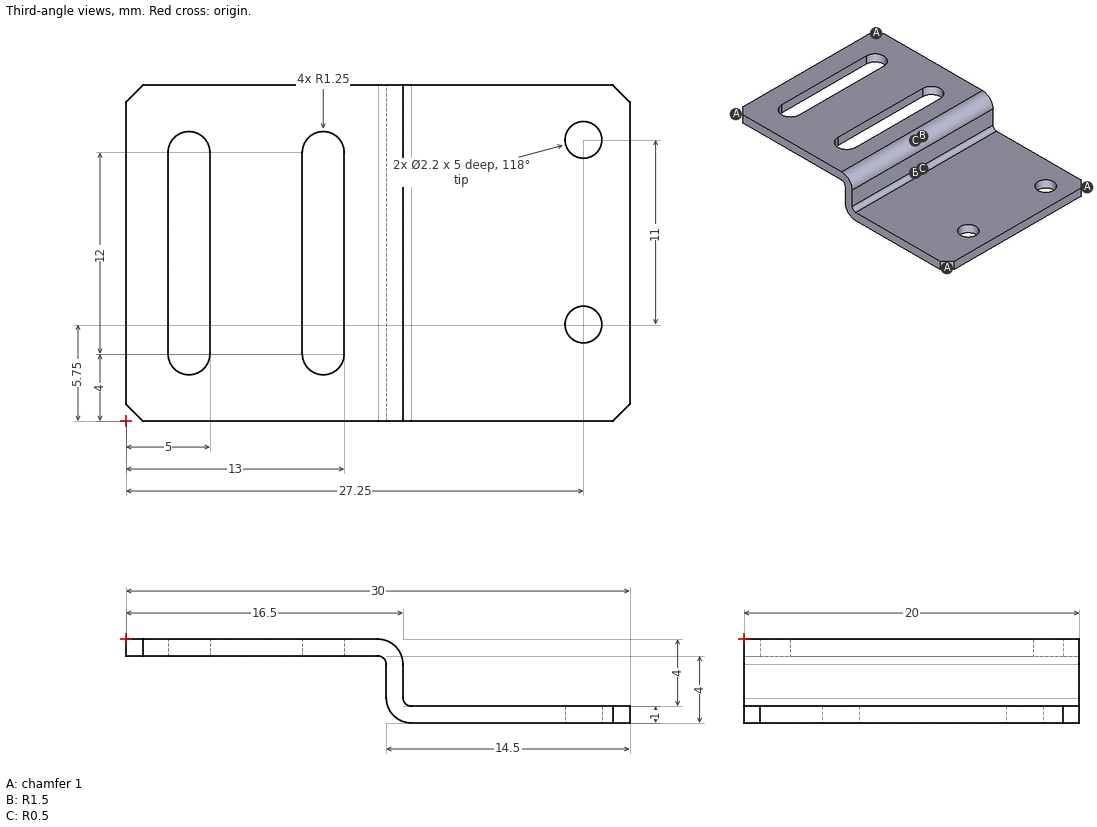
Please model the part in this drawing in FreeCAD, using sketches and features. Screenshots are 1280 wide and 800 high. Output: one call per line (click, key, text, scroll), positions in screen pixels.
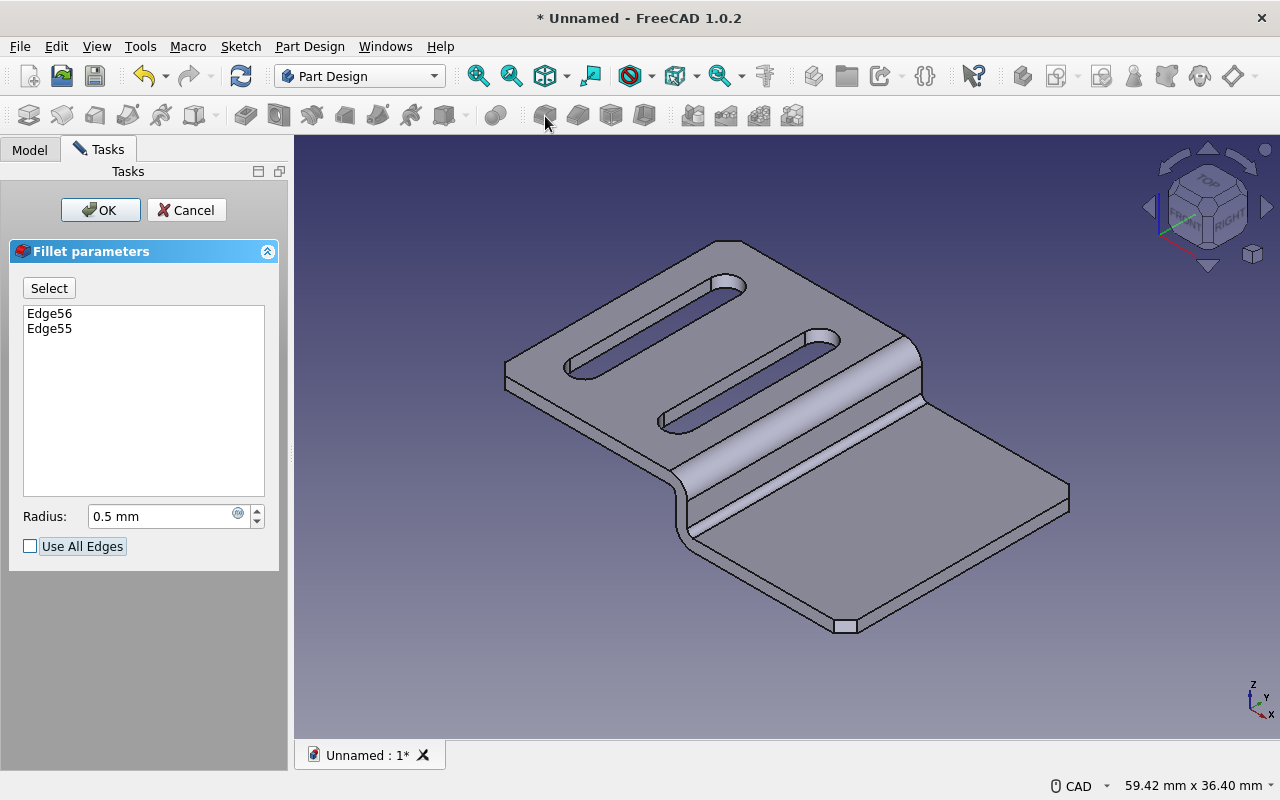
click(101, 210)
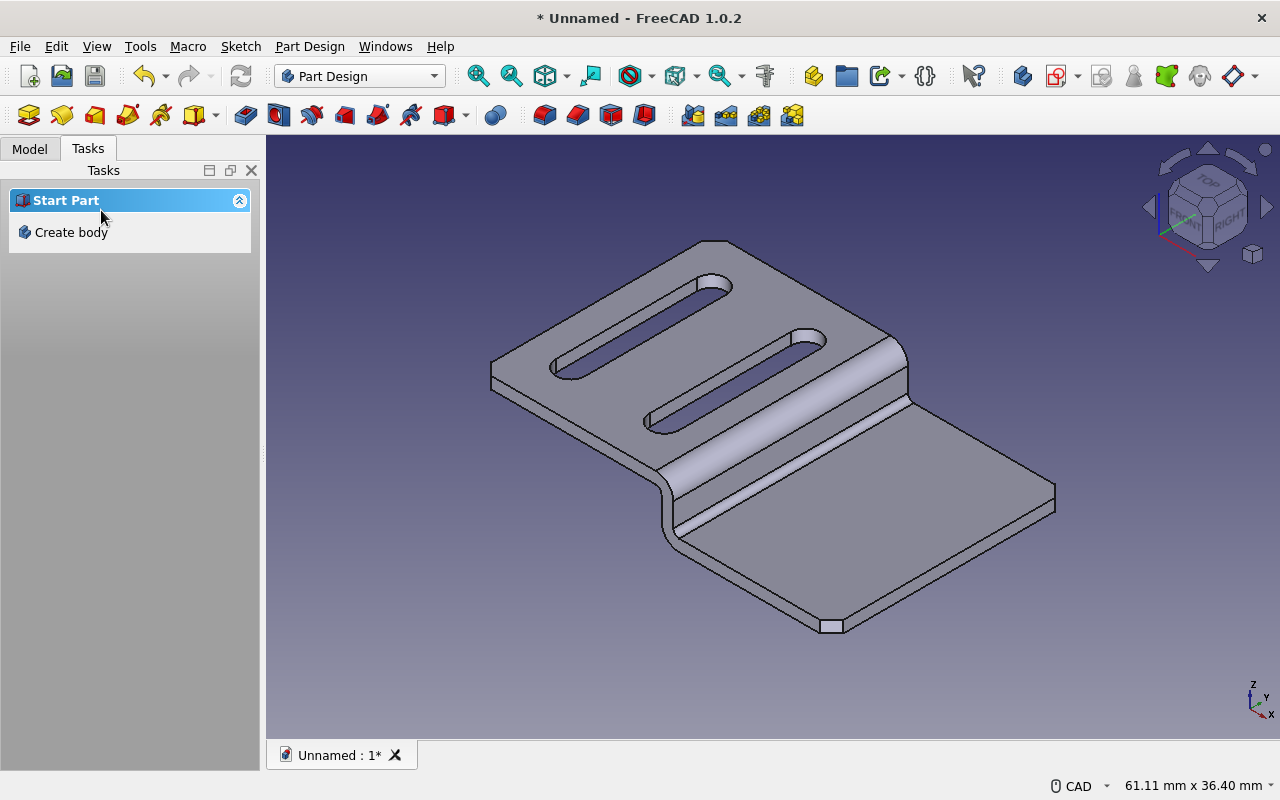
click(906, 495)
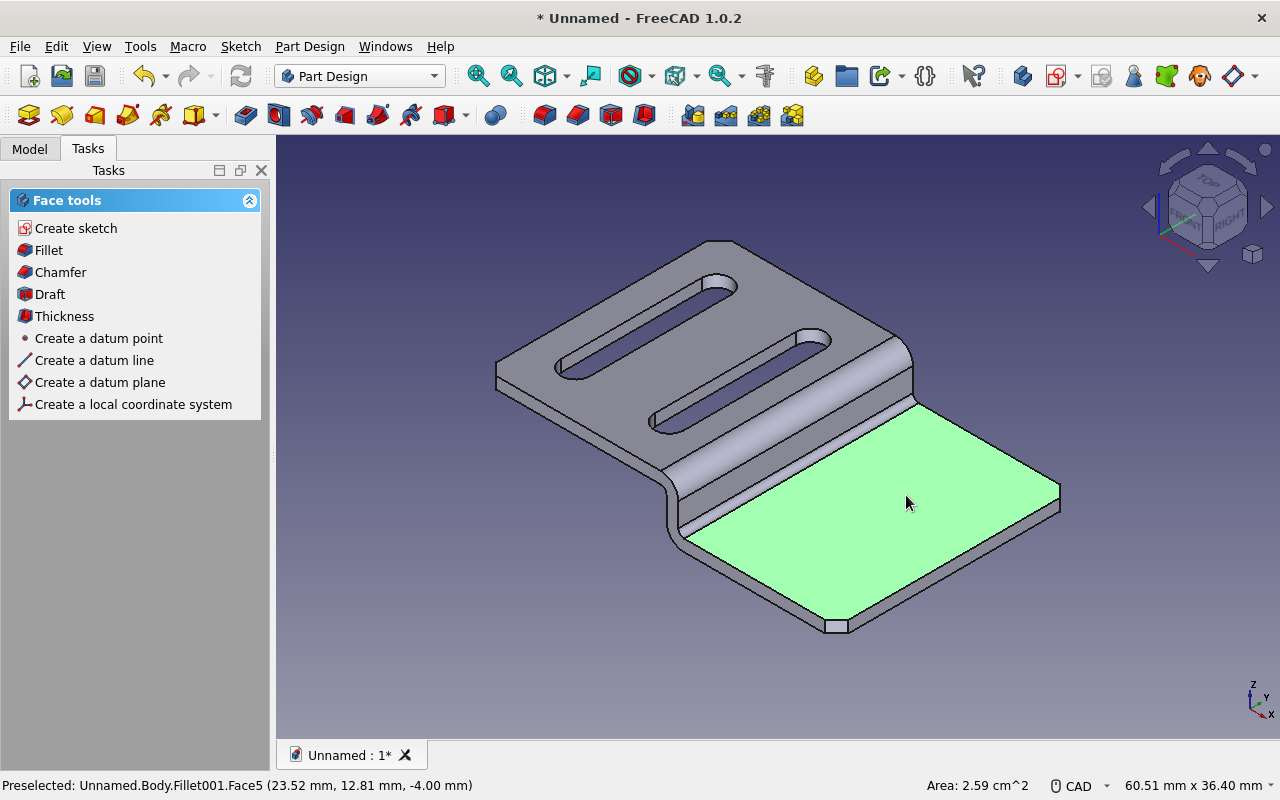
click(1056, 76)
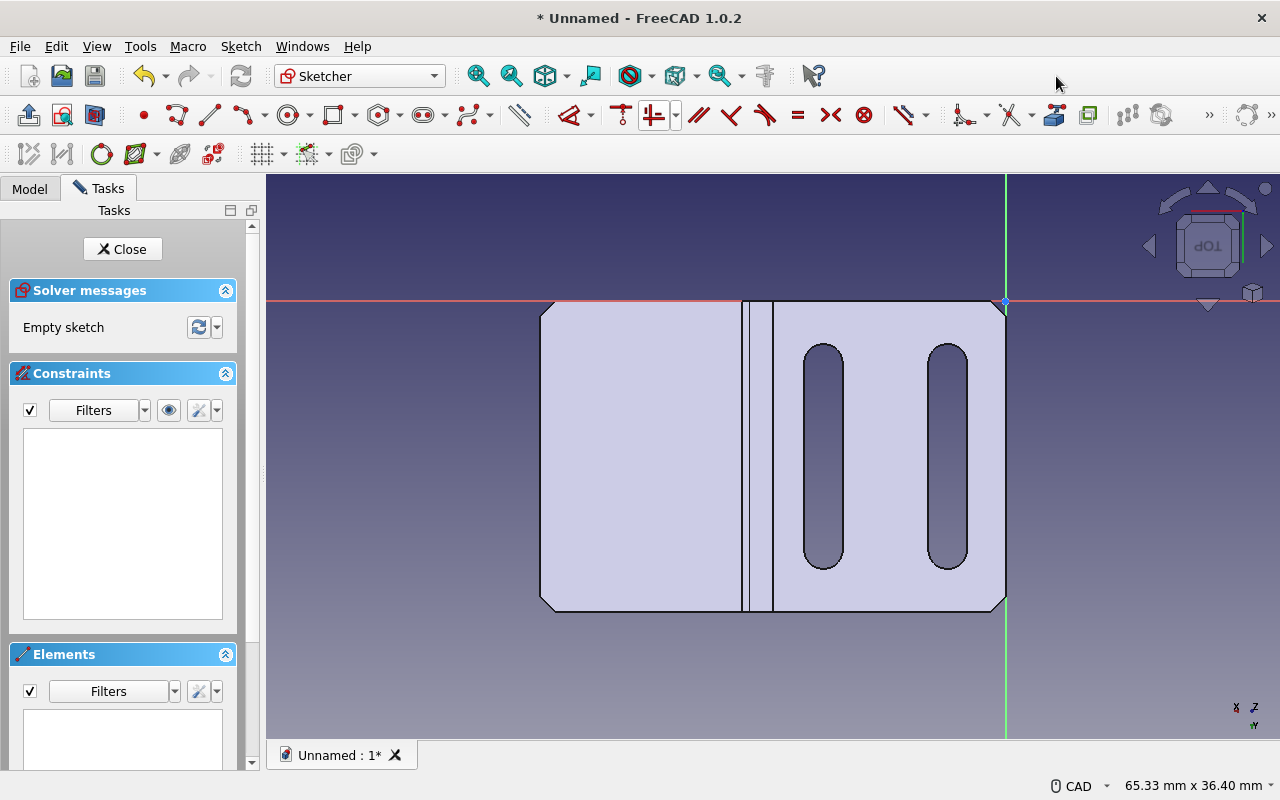
click(95, 116)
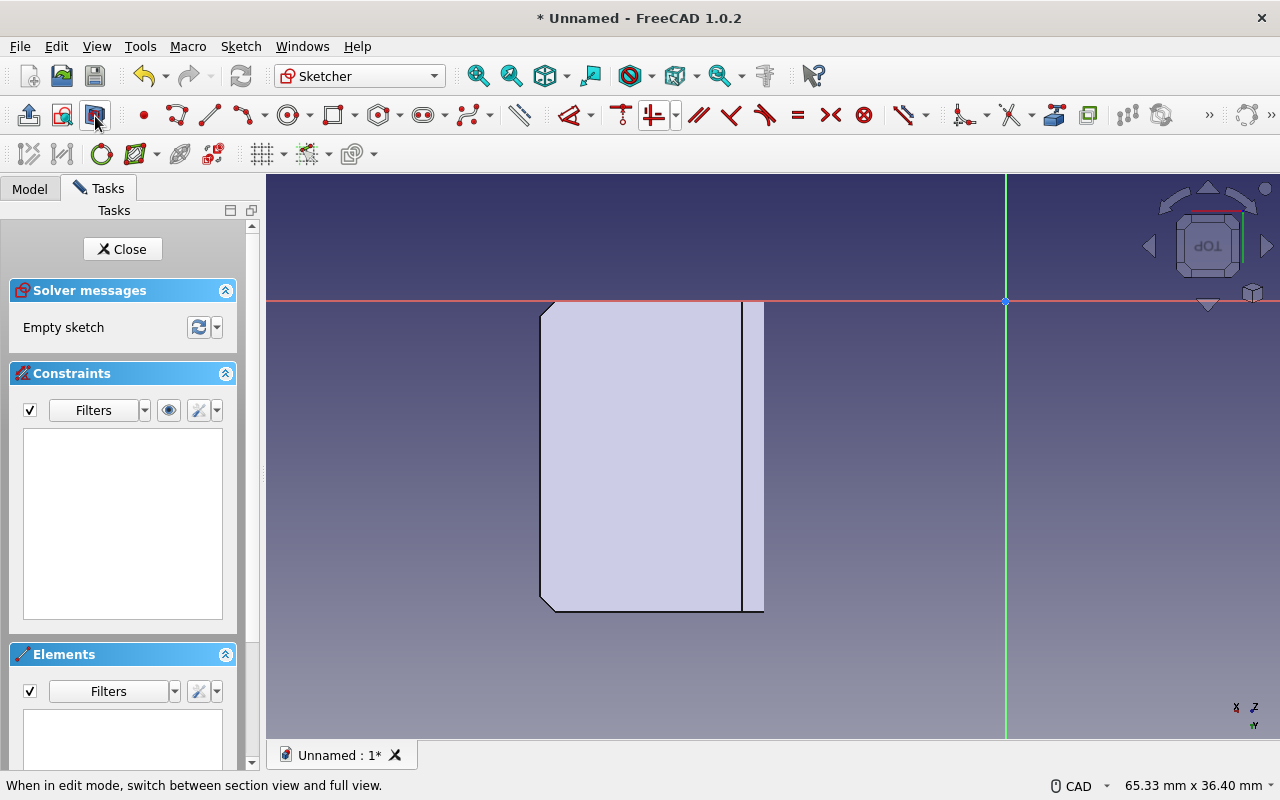
click(288, 116)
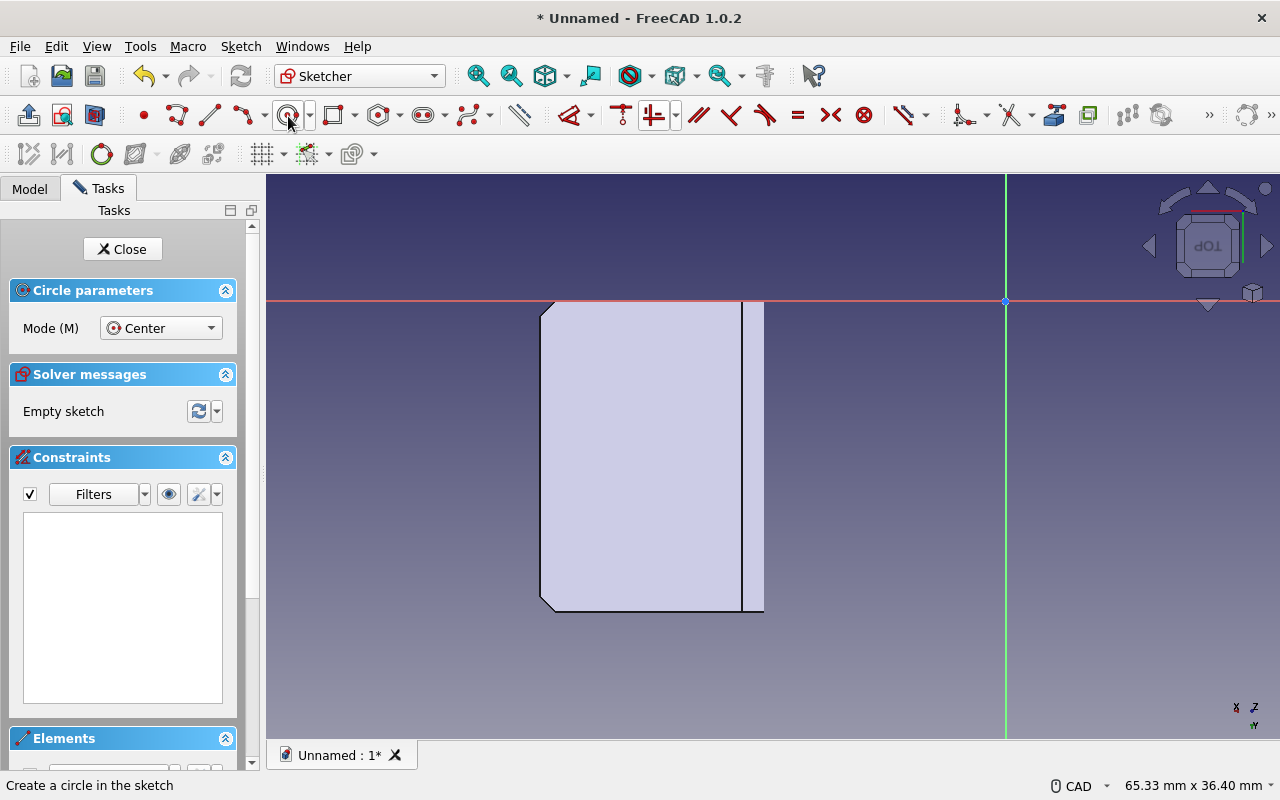
scroll(583, 561, up, 2)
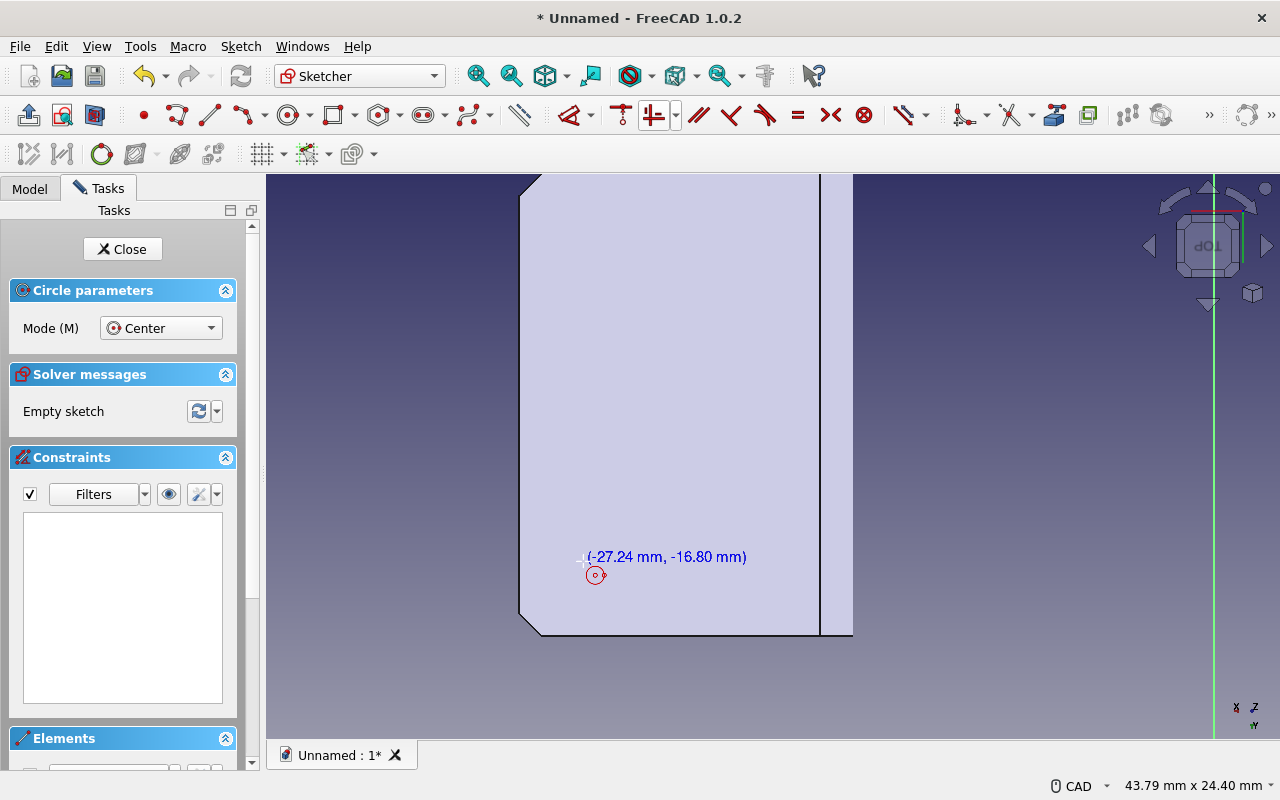
click(583, 561)
click(601, 543)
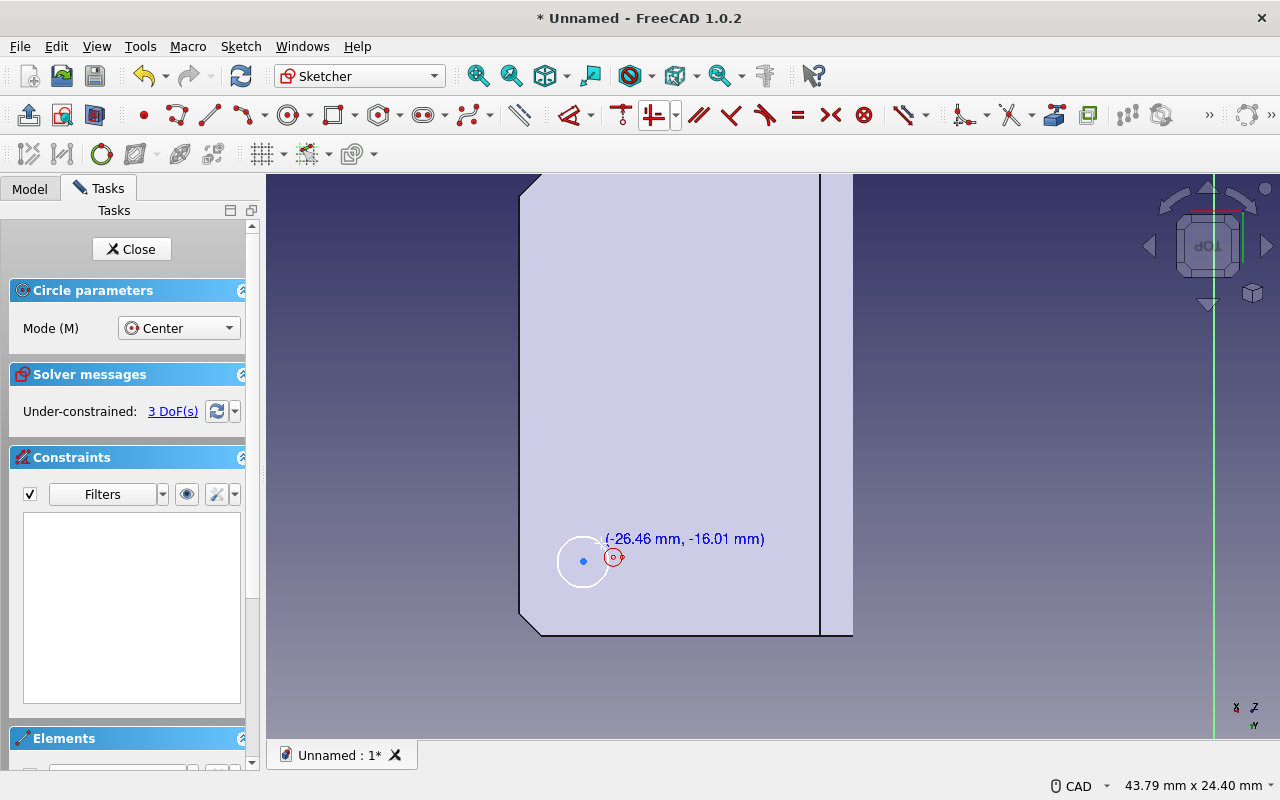
click(583, 306)
click(601, 288)
key(Escape)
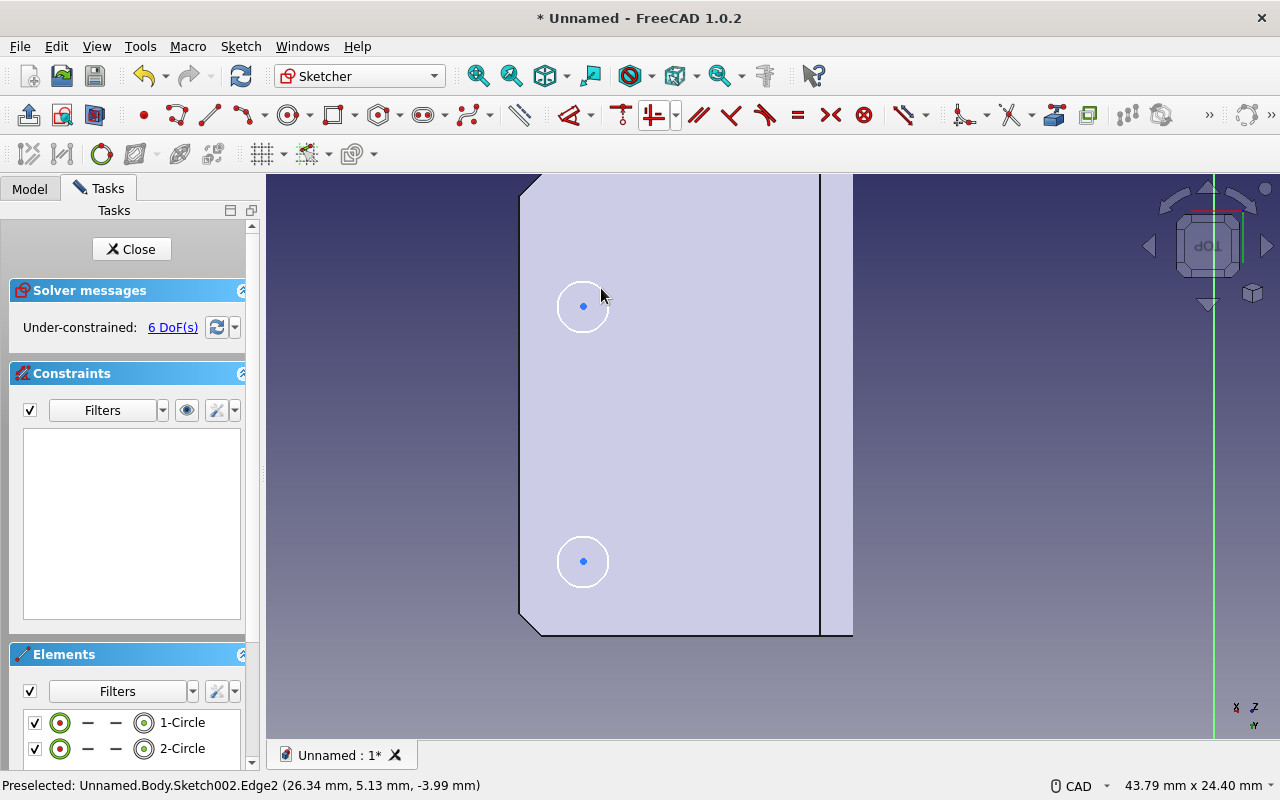
click(601, 544)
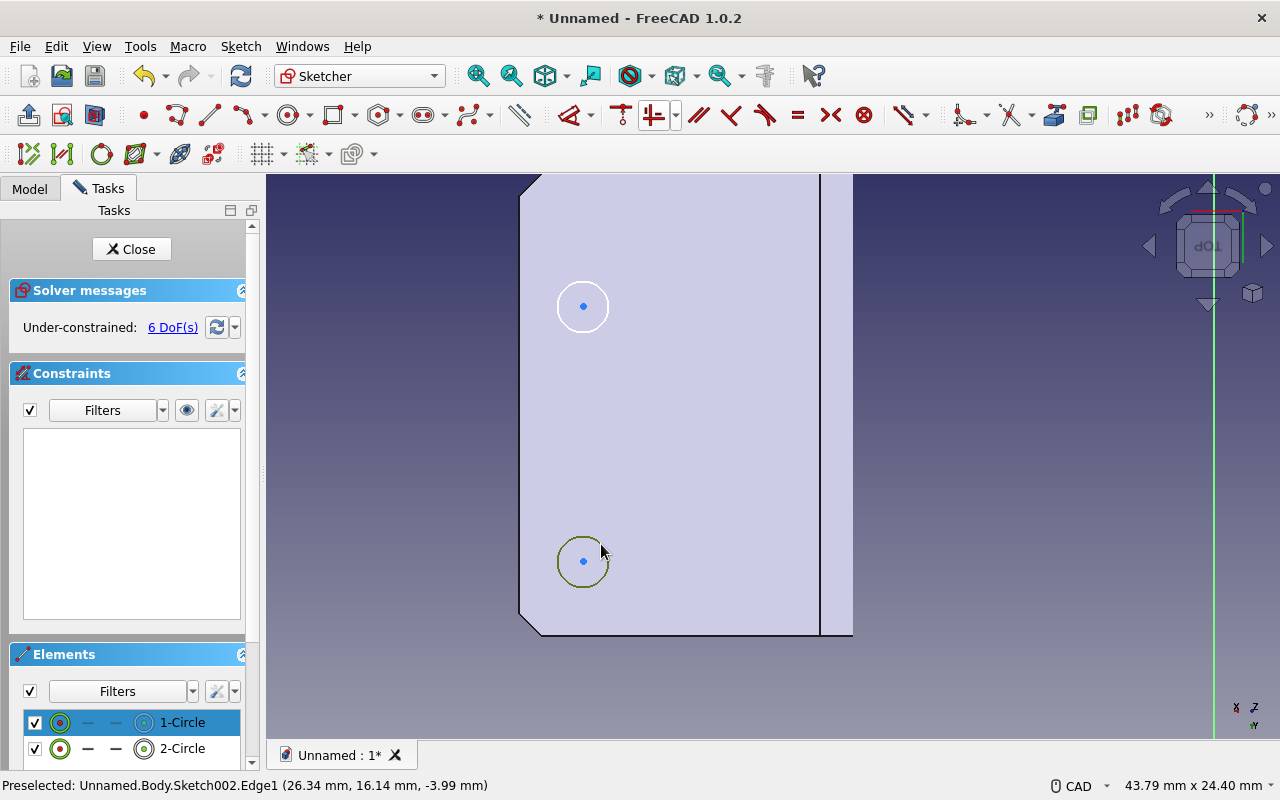
click(601, 289)